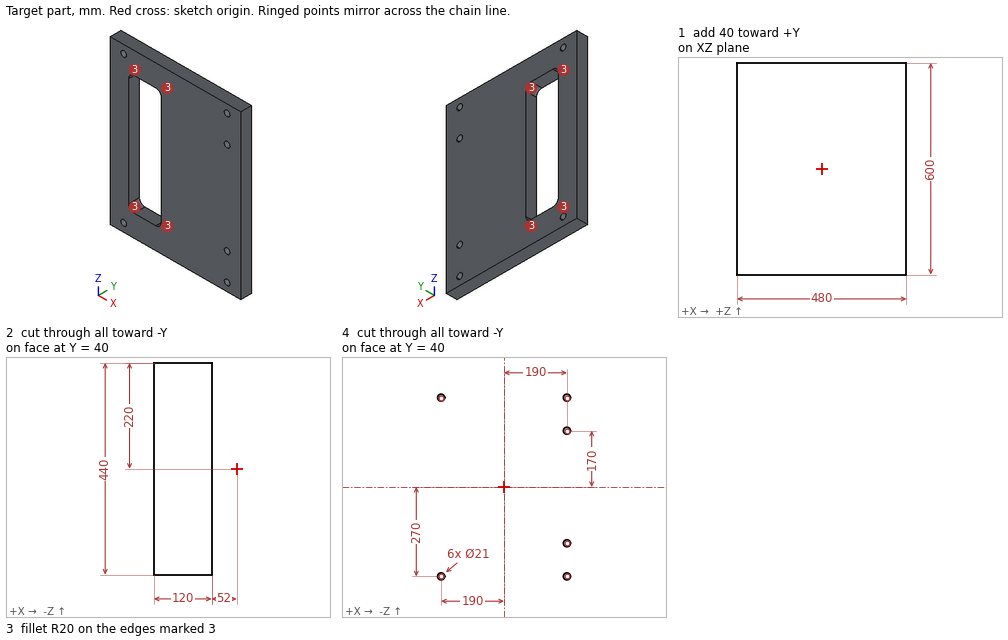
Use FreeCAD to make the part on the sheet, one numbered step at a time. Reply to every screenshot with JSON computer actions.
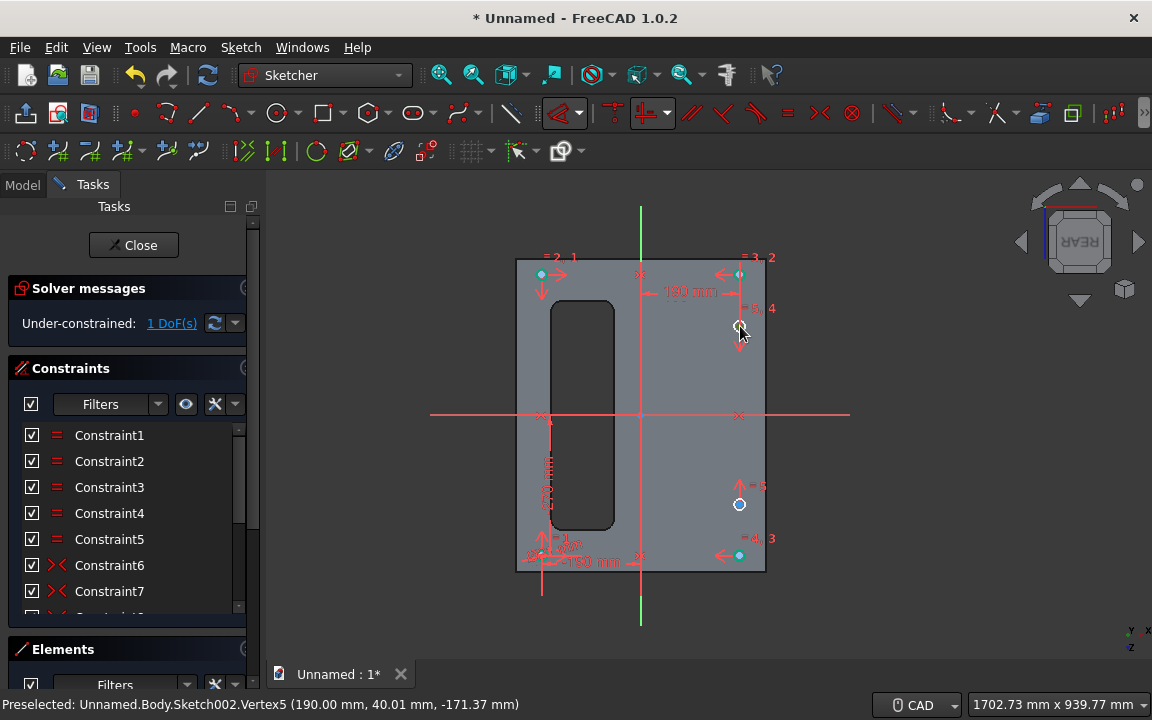
{"action": "key", "text": "i"}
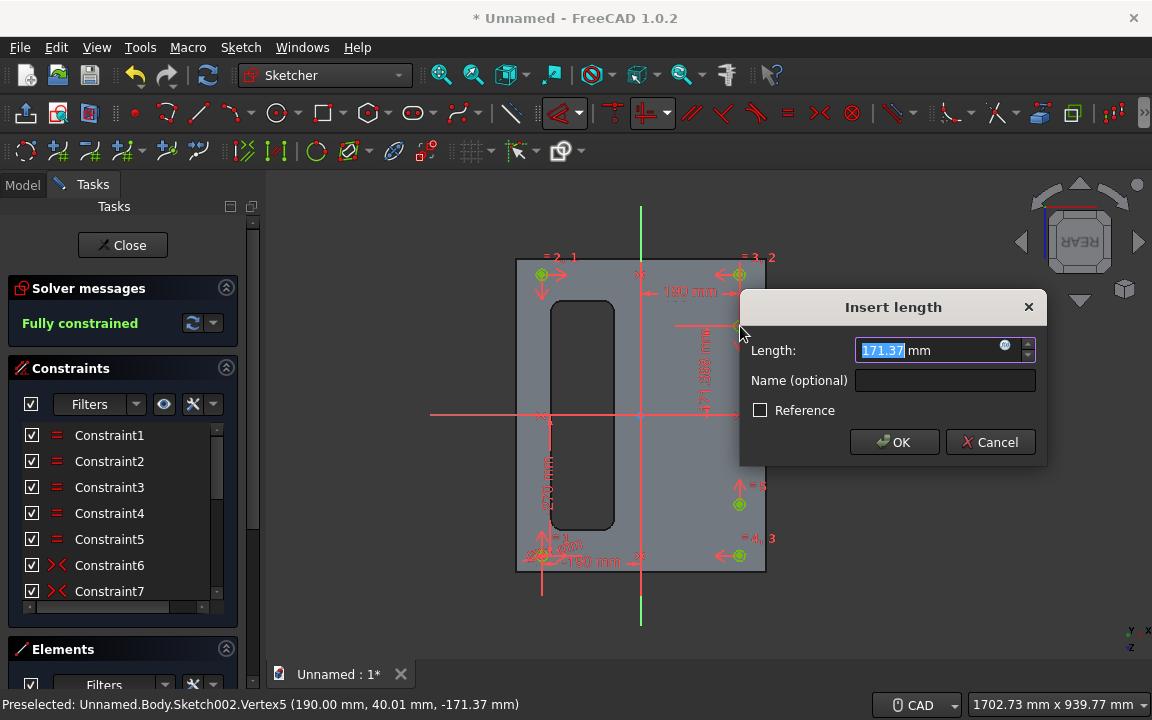
{"action": "type", "text": "170"}
{"action": "key", "text": "Return"}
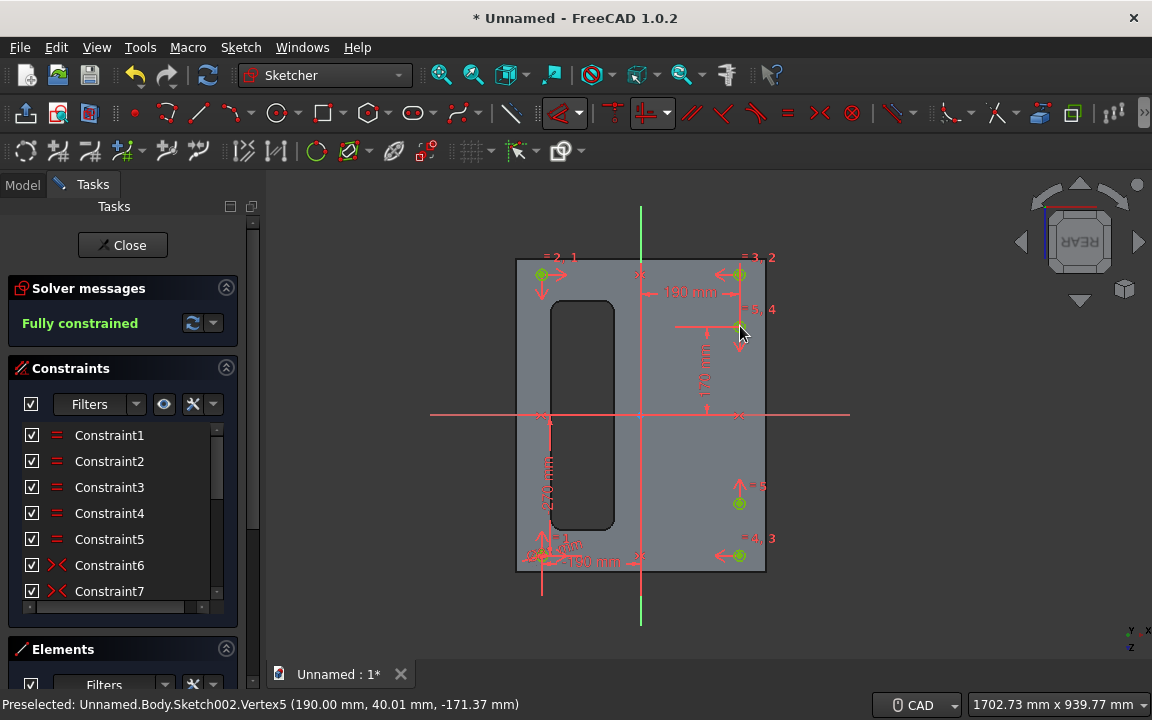
{"action": "left_click", "coordinate": [123, 245]}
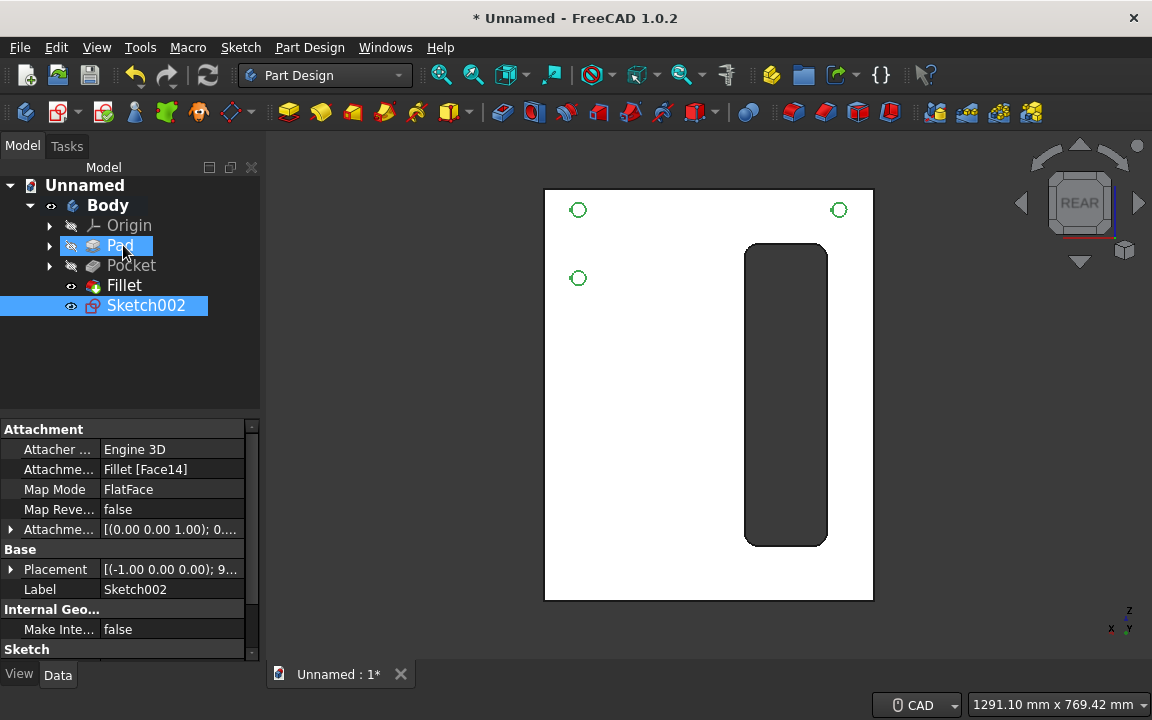
{"action": "left_click", "coordinate": [504, 112]}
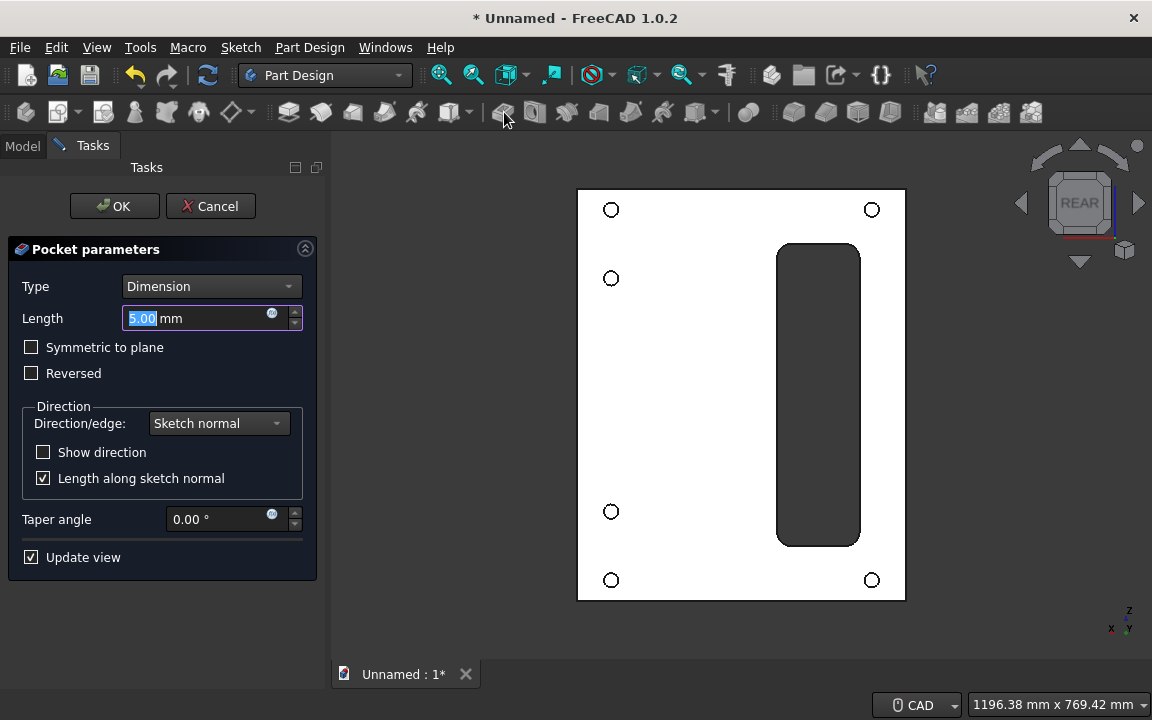
{"action": "left_click", "coordinate": [212, 286]}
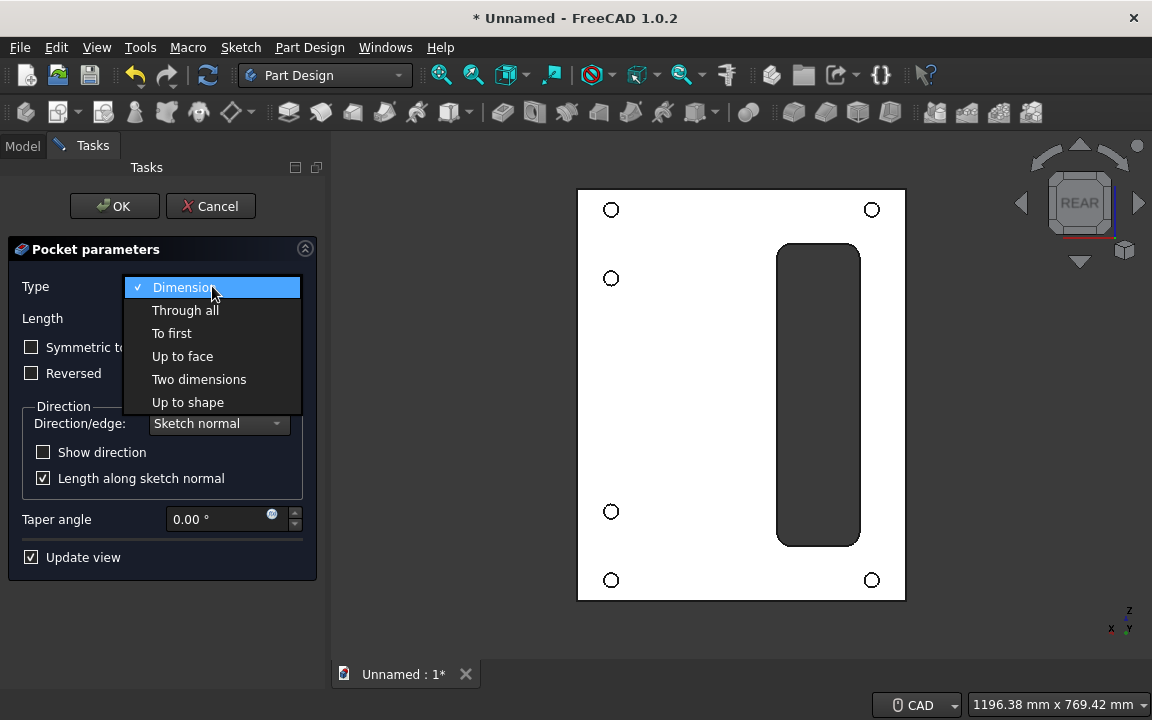
{"action": "left_click", "coordinate": [212, 310]}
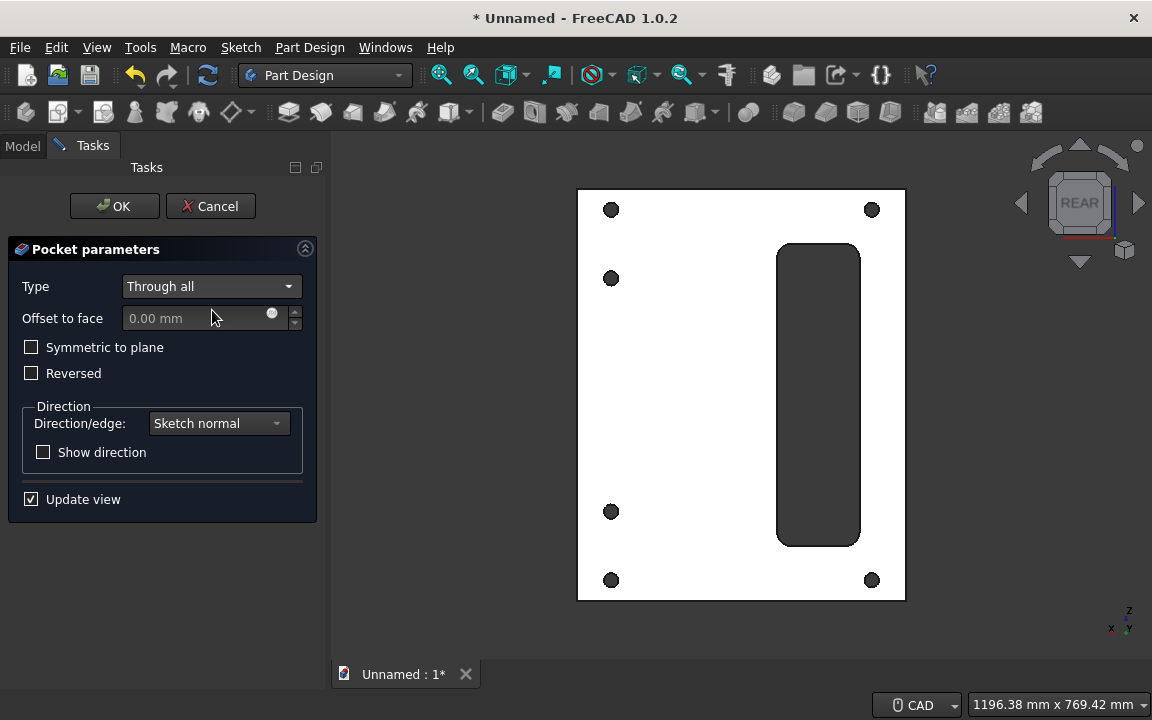
{"action": "left_click", "coordinate": [115, 206]}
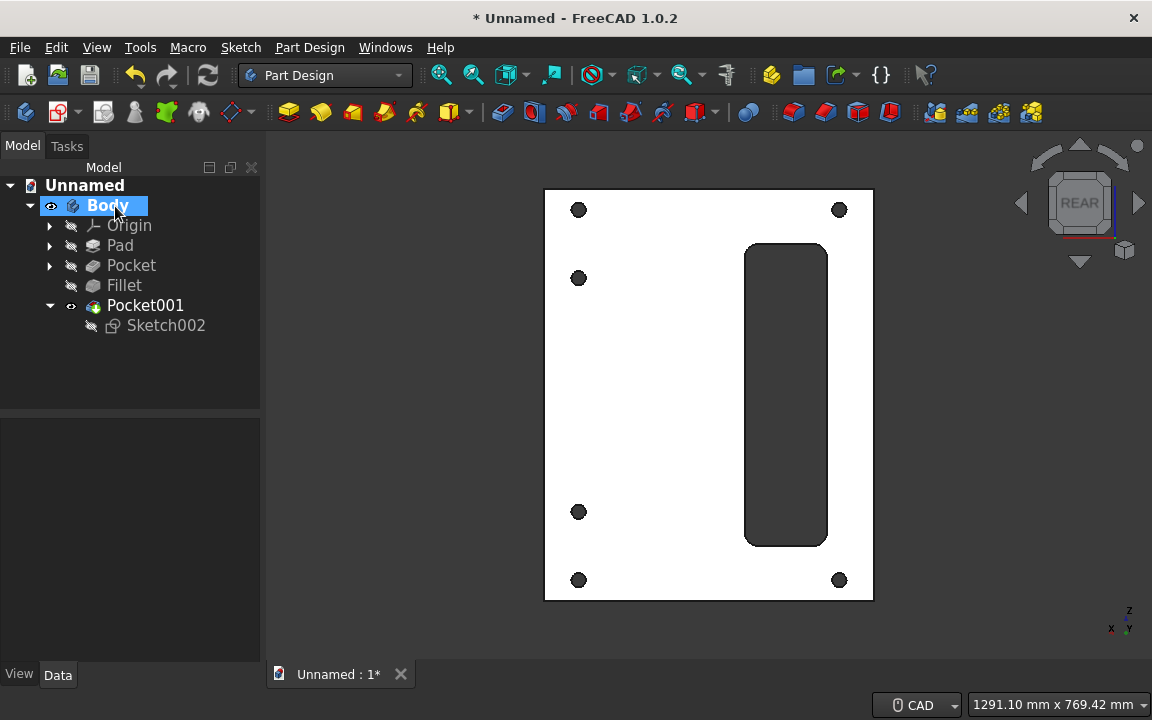
{"action": "key", "text": "0"}